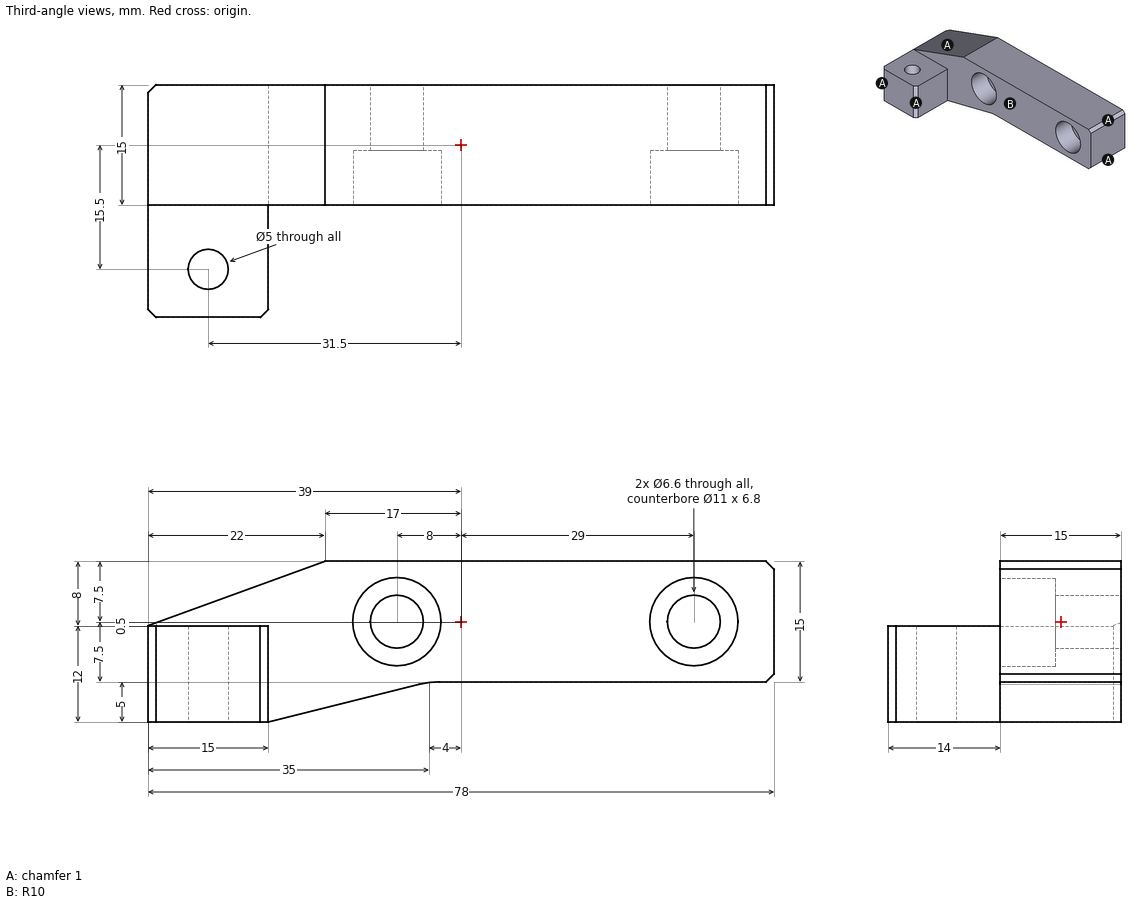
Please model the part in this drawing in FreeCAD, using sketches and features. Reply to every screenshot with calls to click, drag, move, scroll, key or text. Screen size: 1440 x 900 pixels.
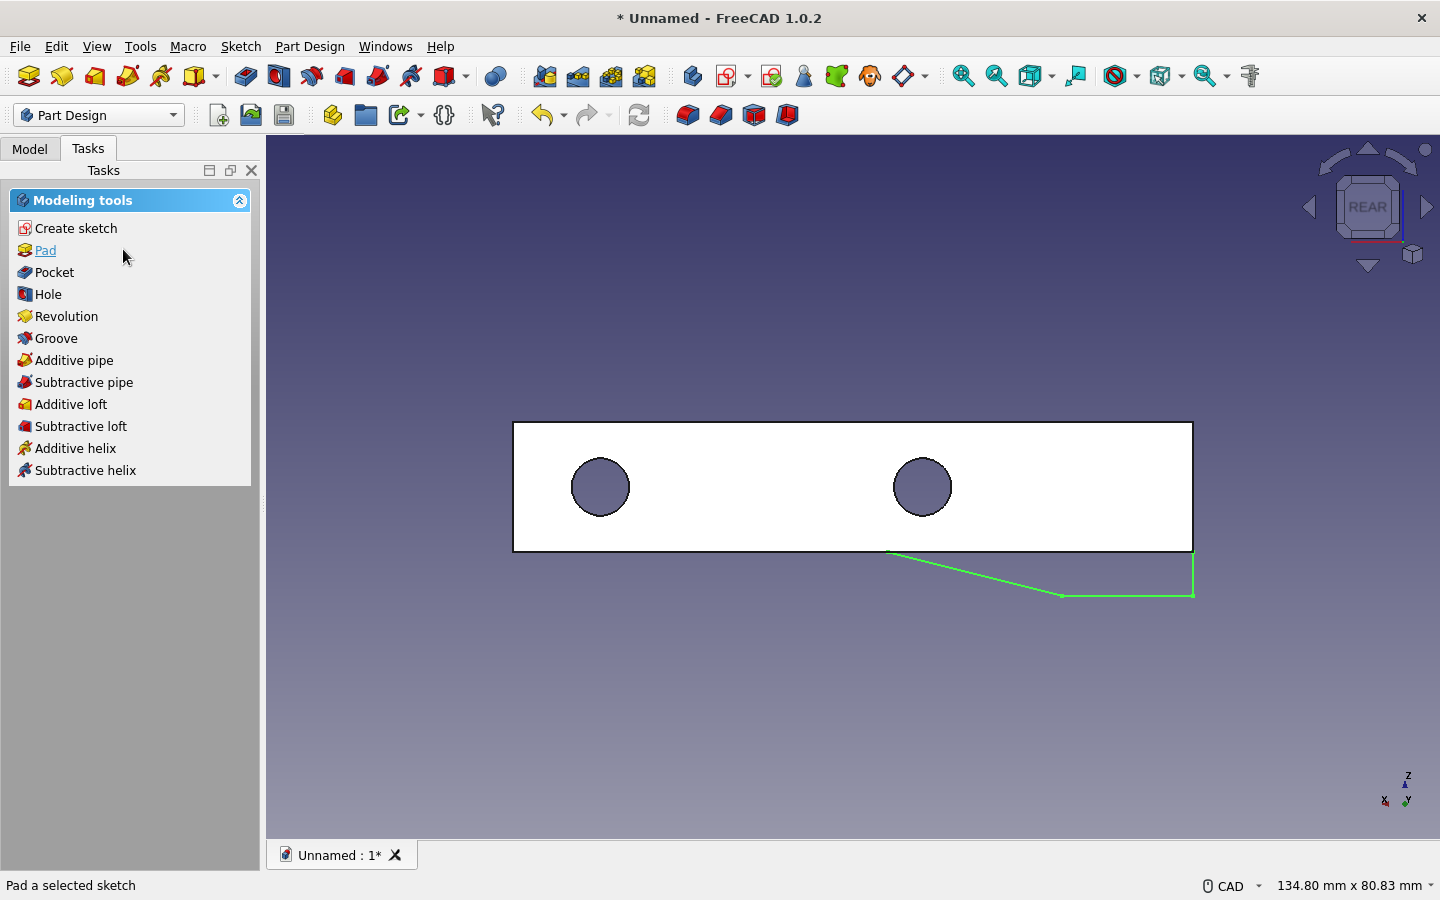
click(29, 76)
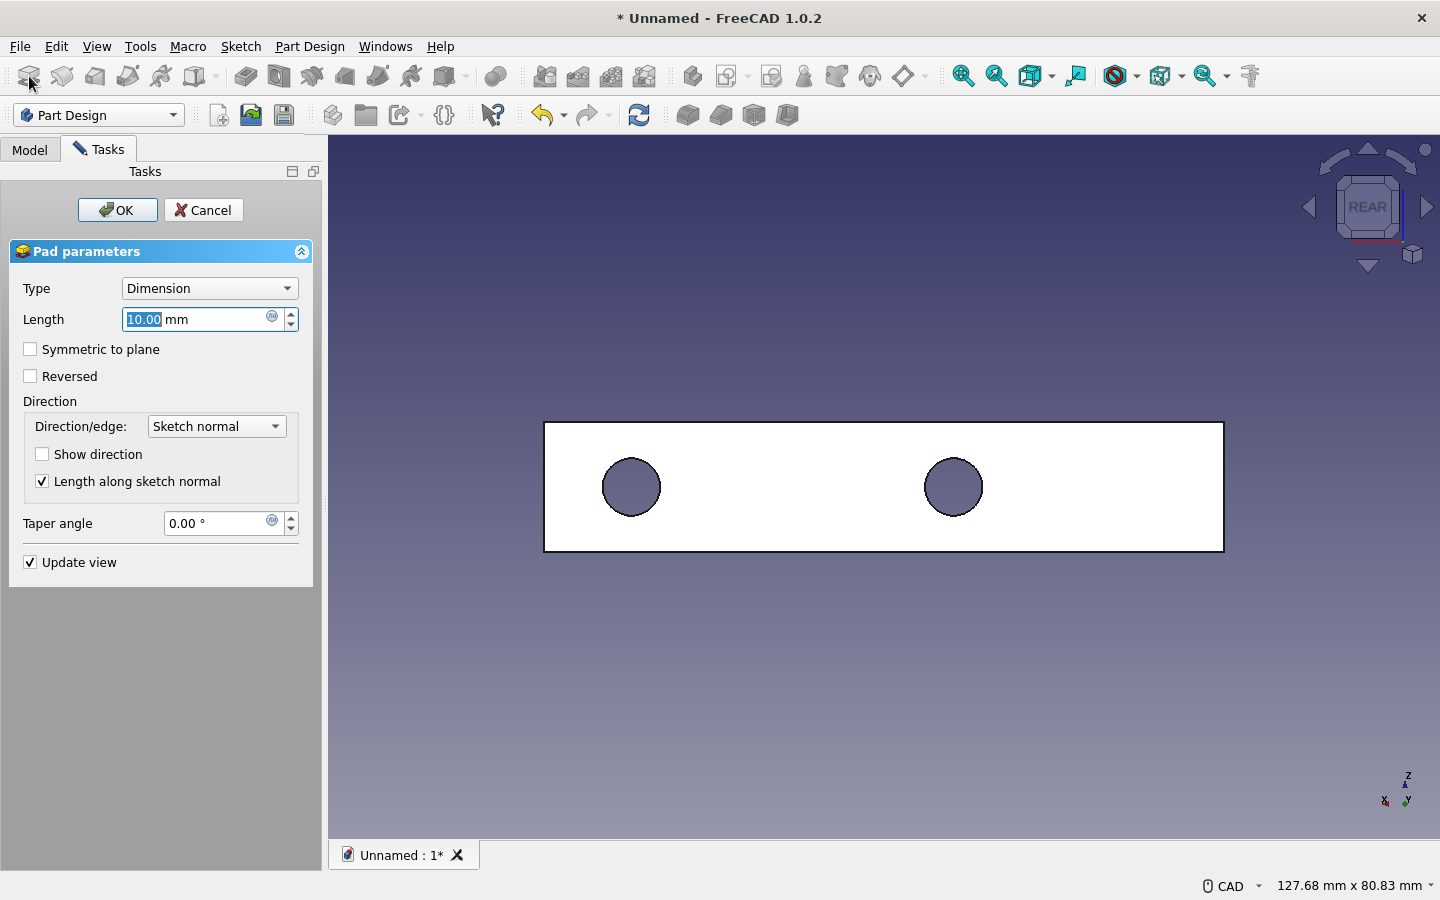
text(15)
key(Tab)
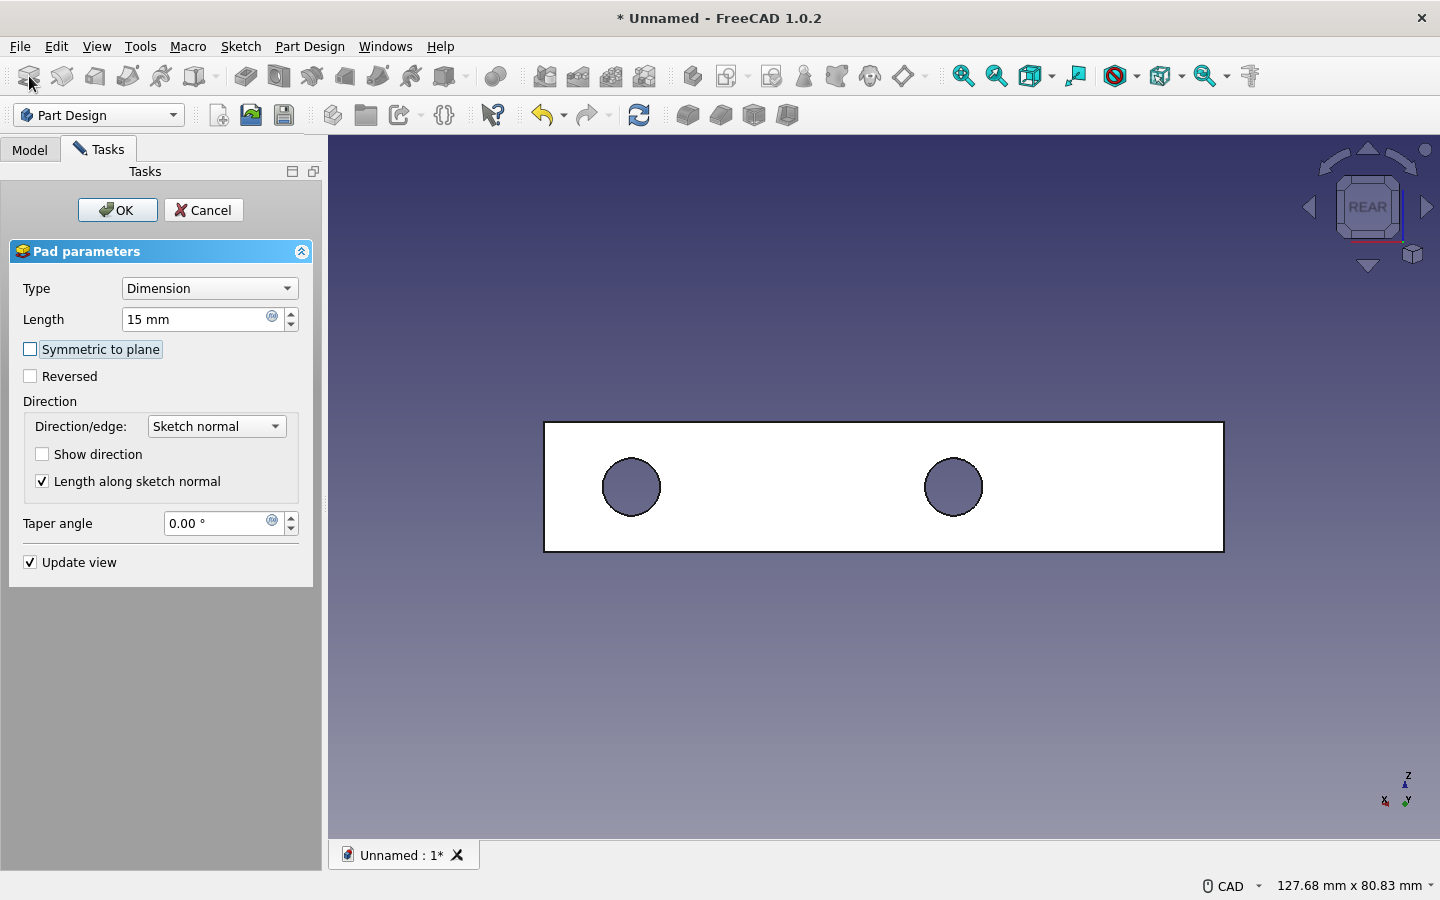
click(31, 376)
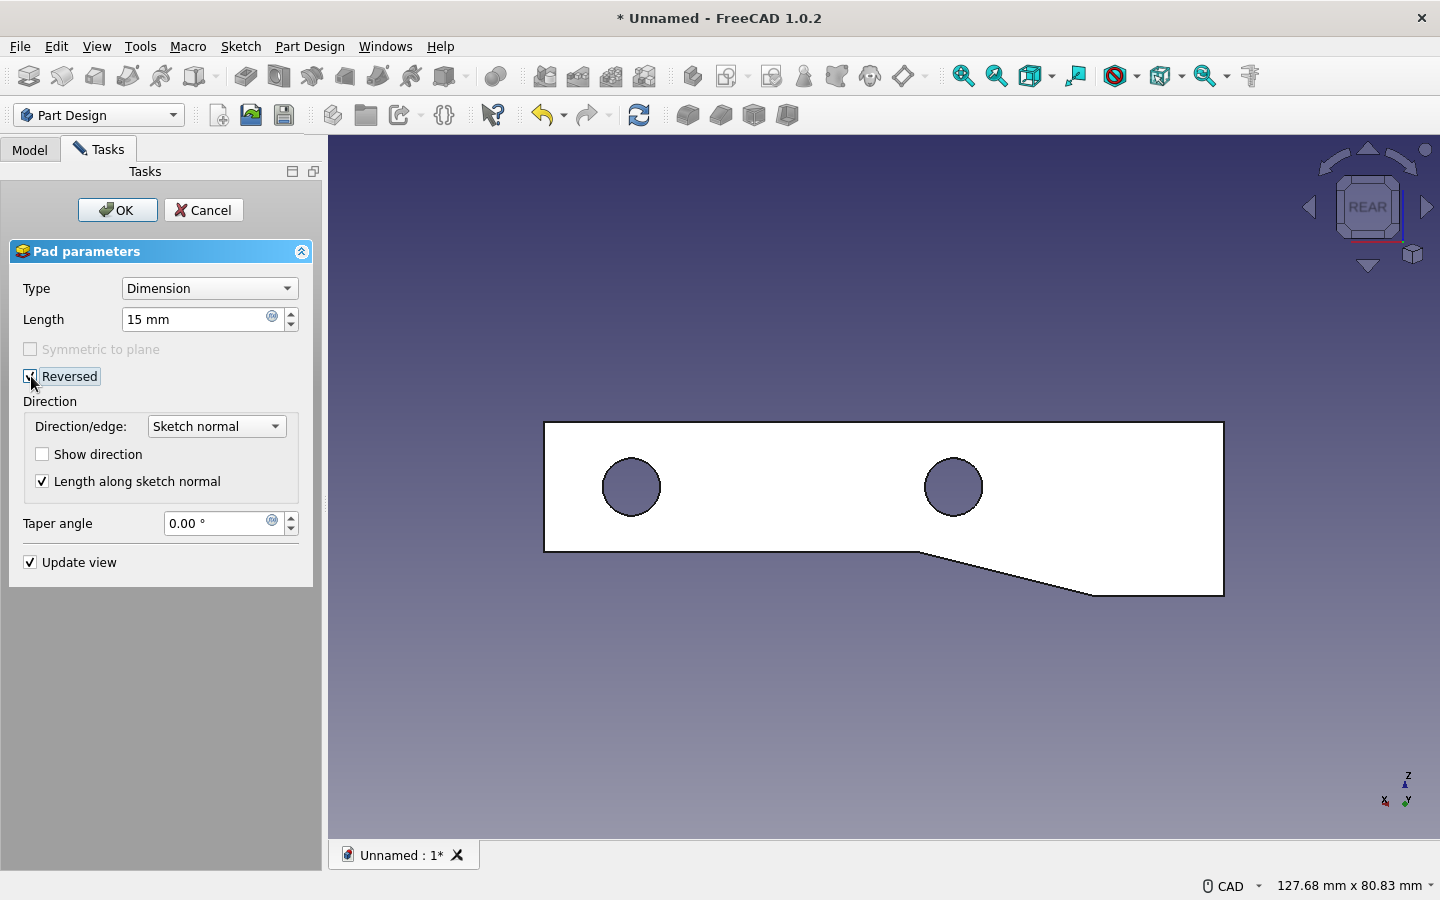
click(118, 210)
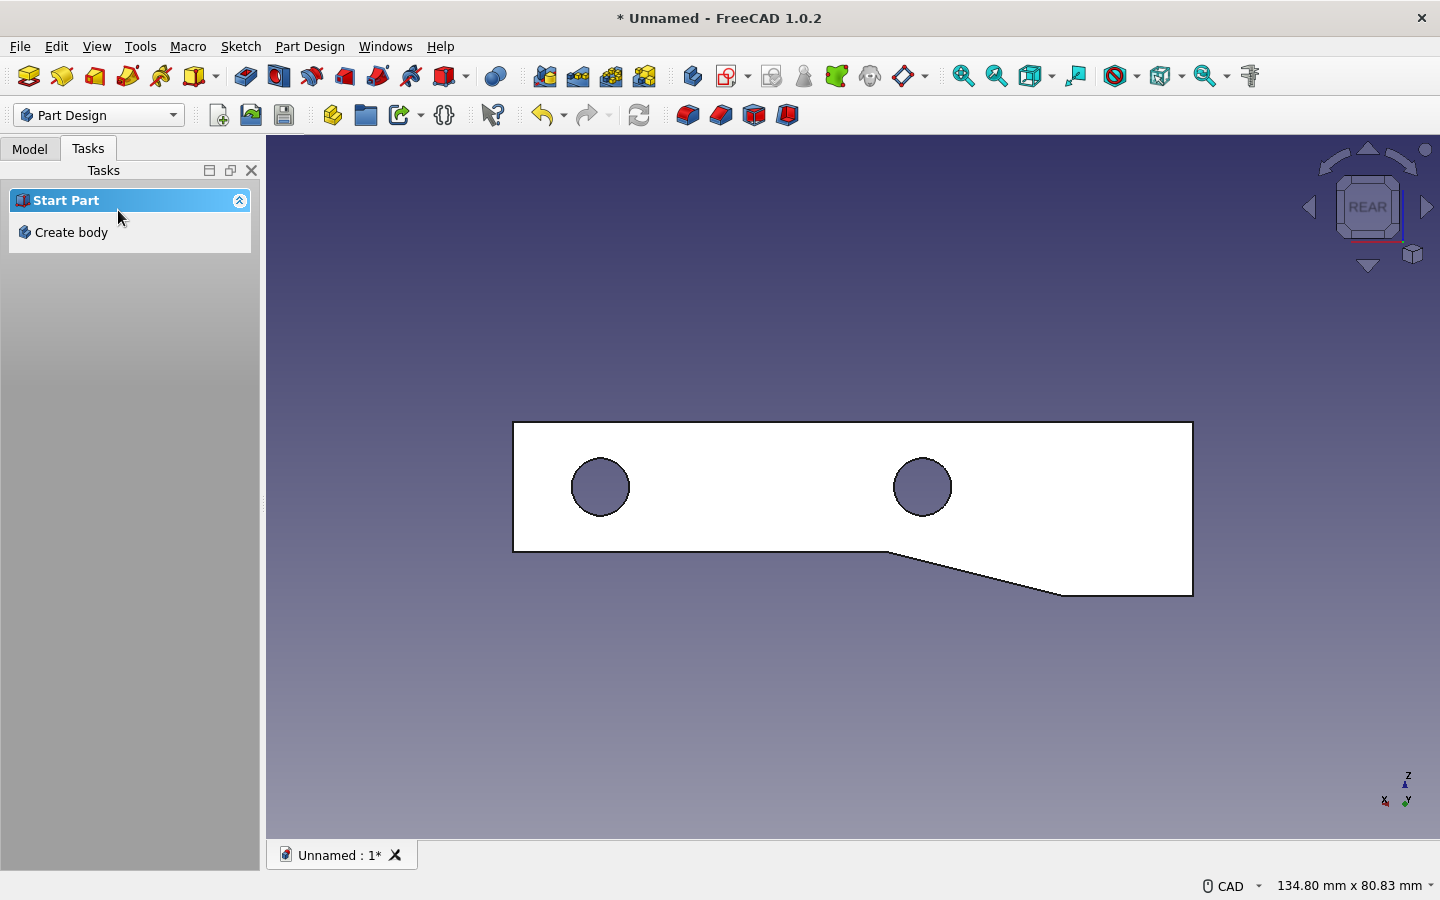
key(0)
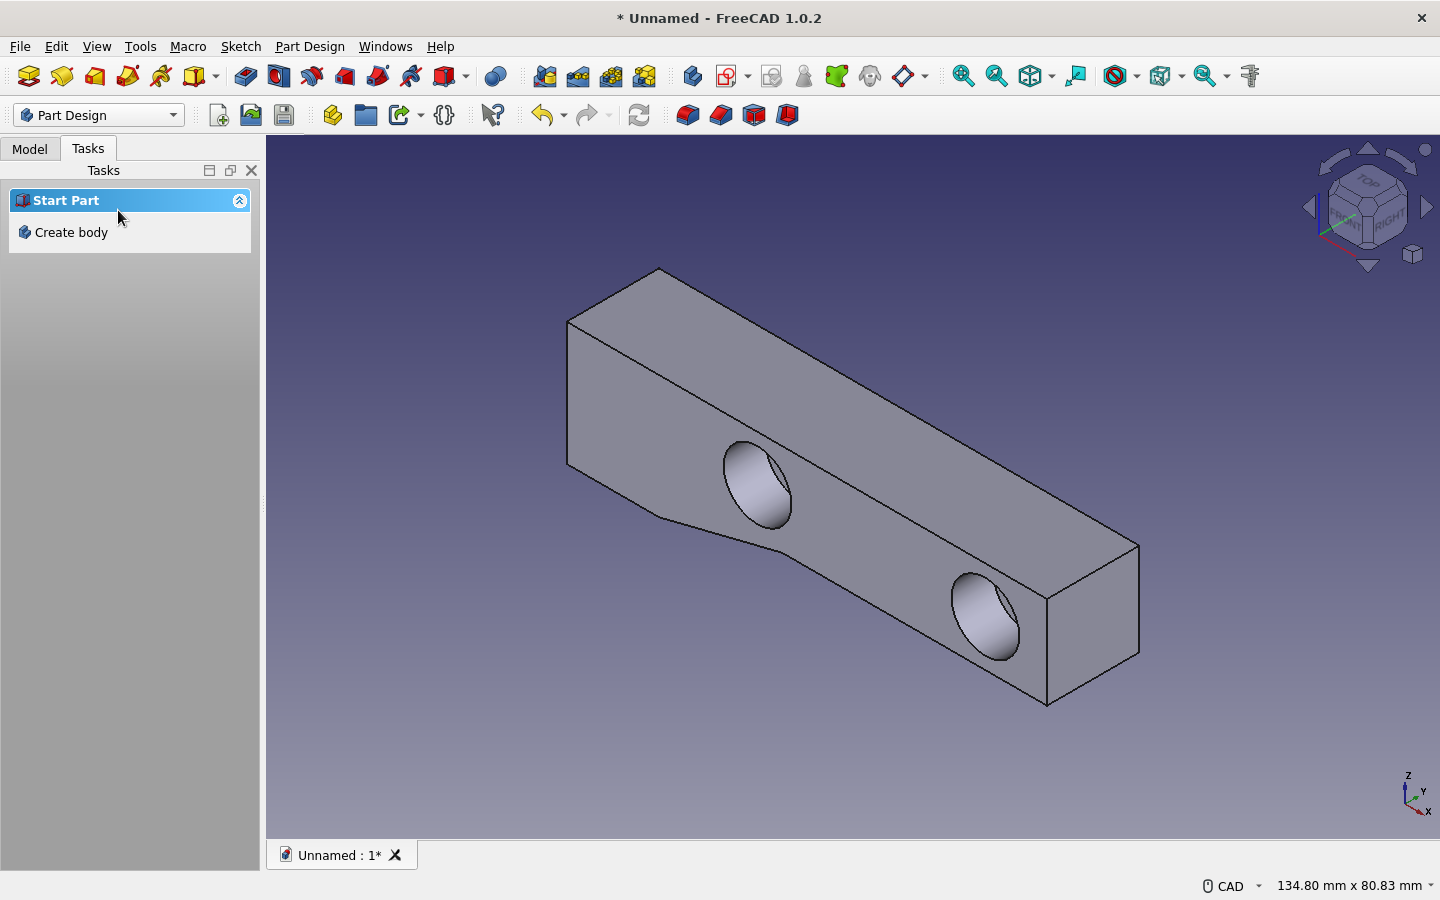
click(670, 451)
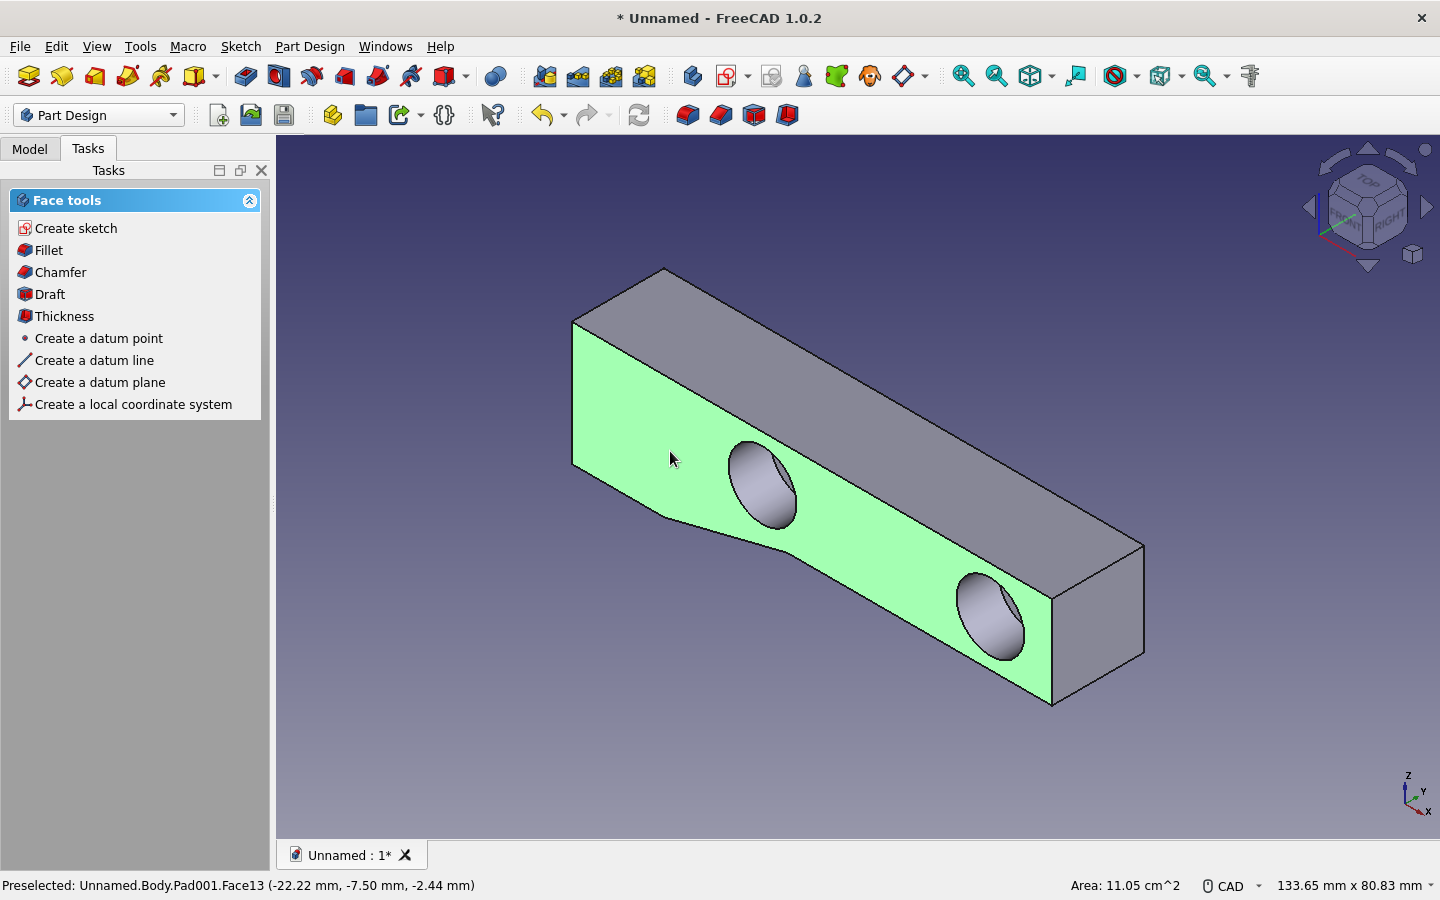
click(726, 76)